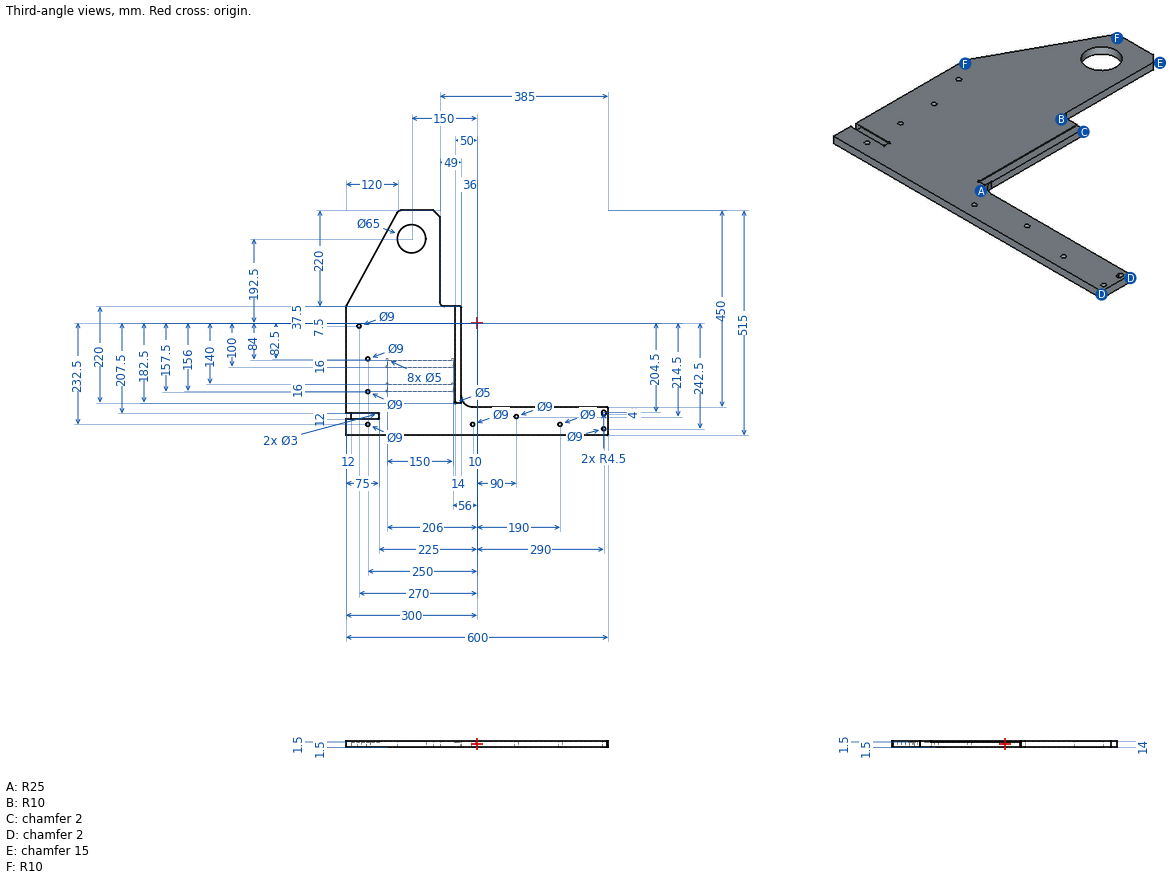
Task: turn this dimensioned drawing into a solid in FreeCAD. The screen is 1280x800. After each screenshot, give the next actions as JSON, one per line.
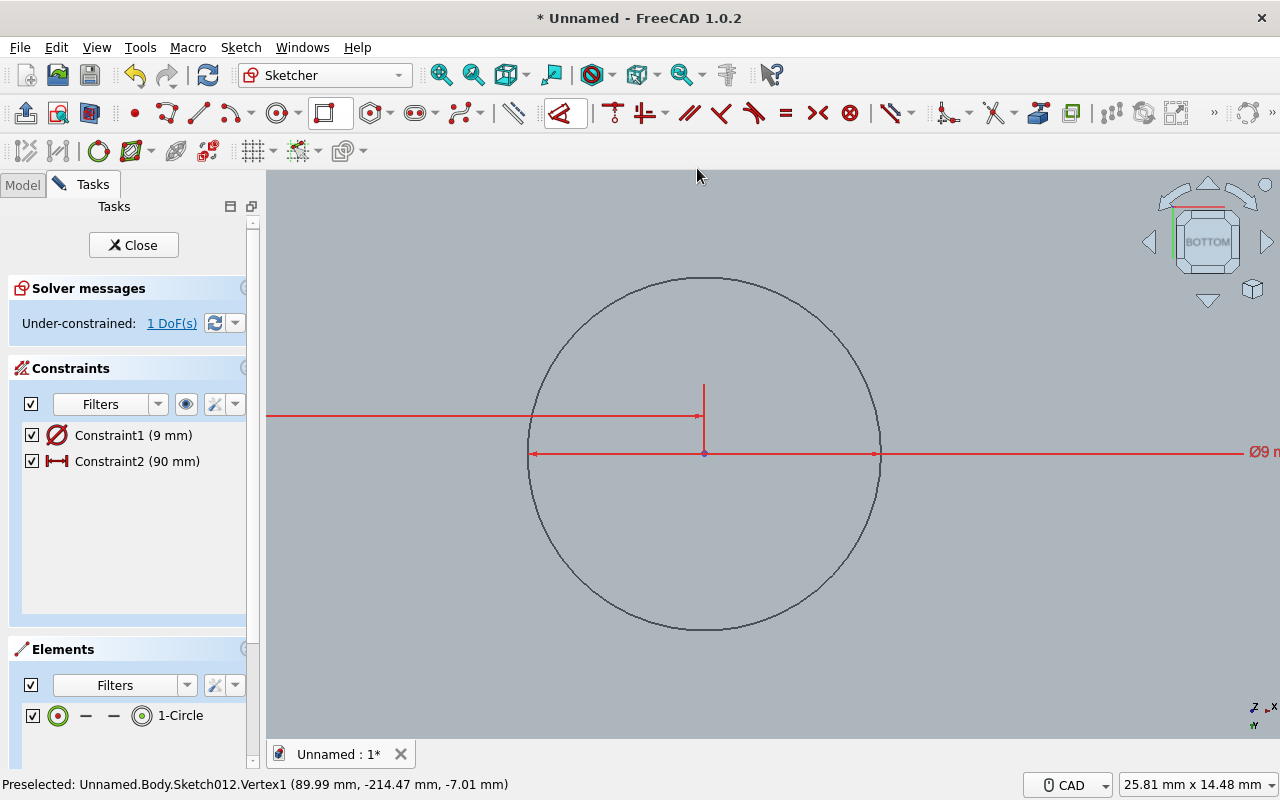
{"action": "left_click", "coordinate": [704, 454]}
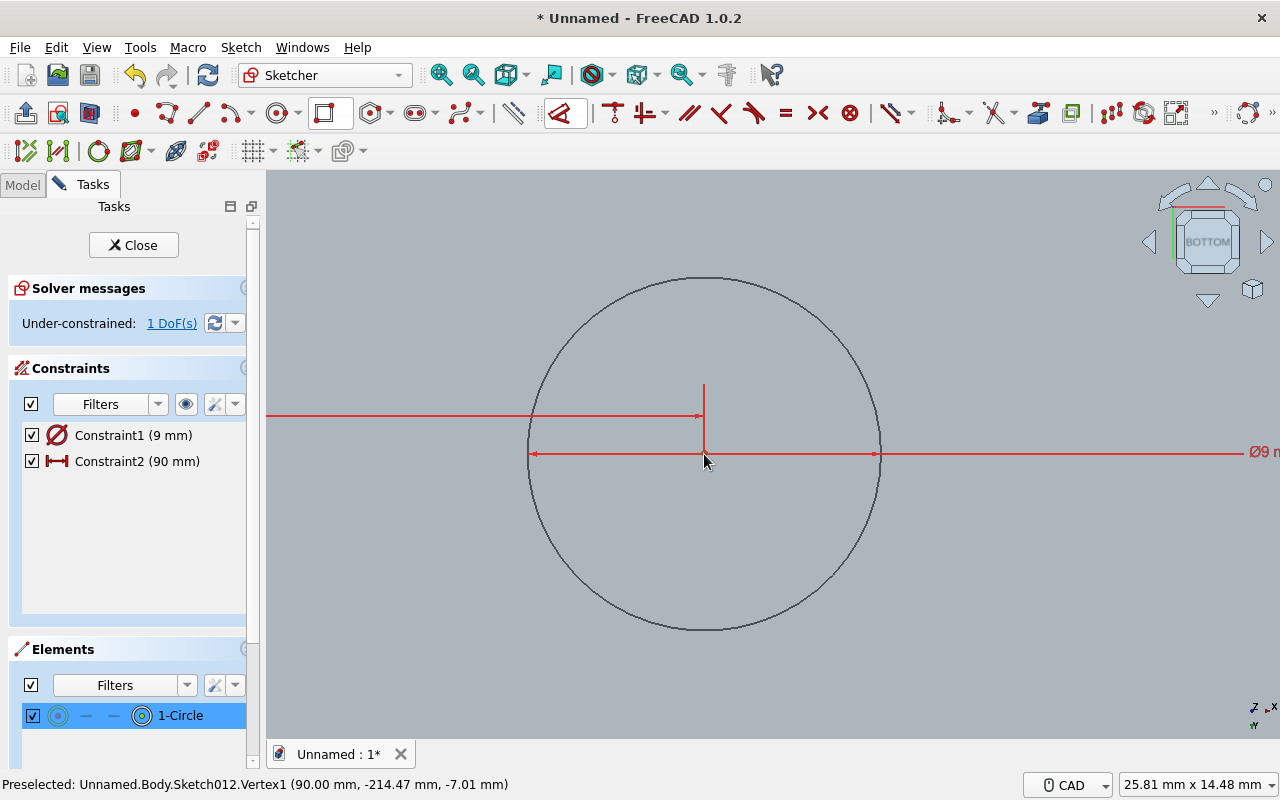
{"action": "left_click", "coordinate": [582, 114]}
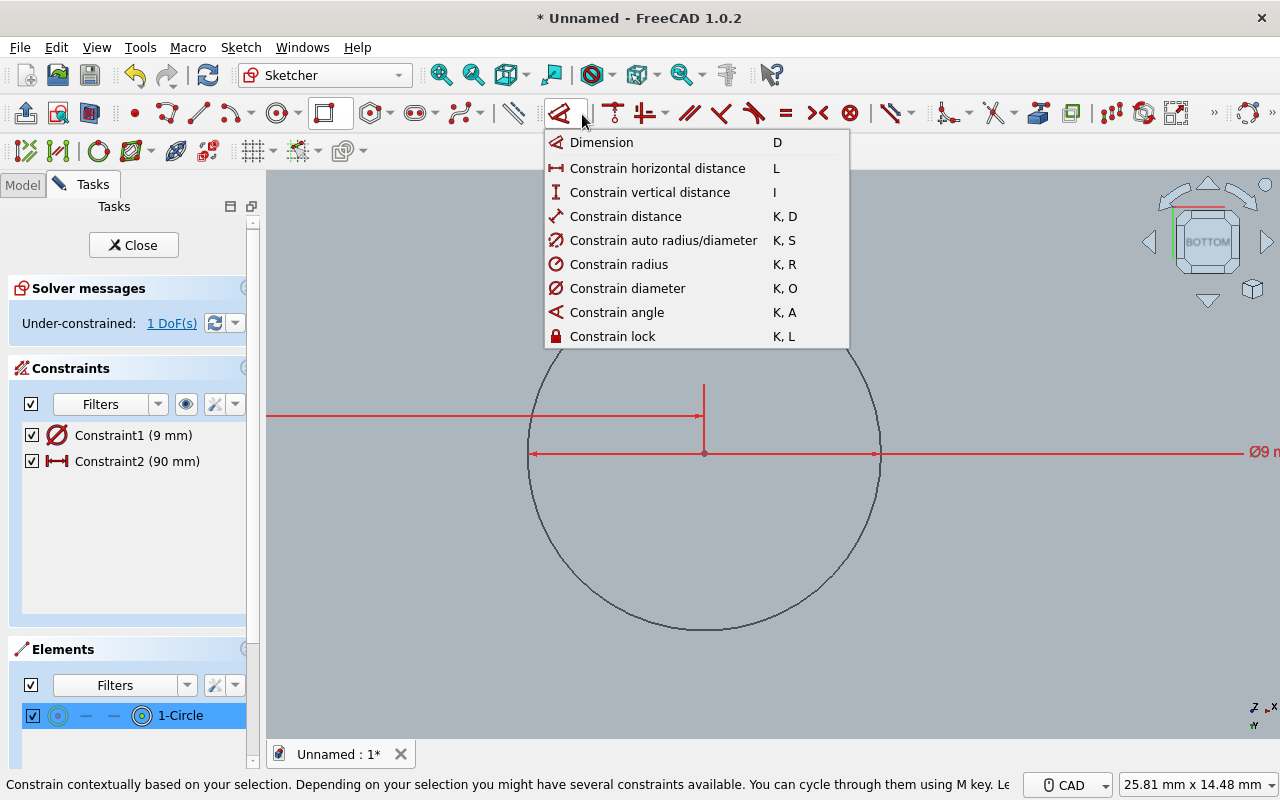
{"action": "left_click", "coordinate": [697, 192]}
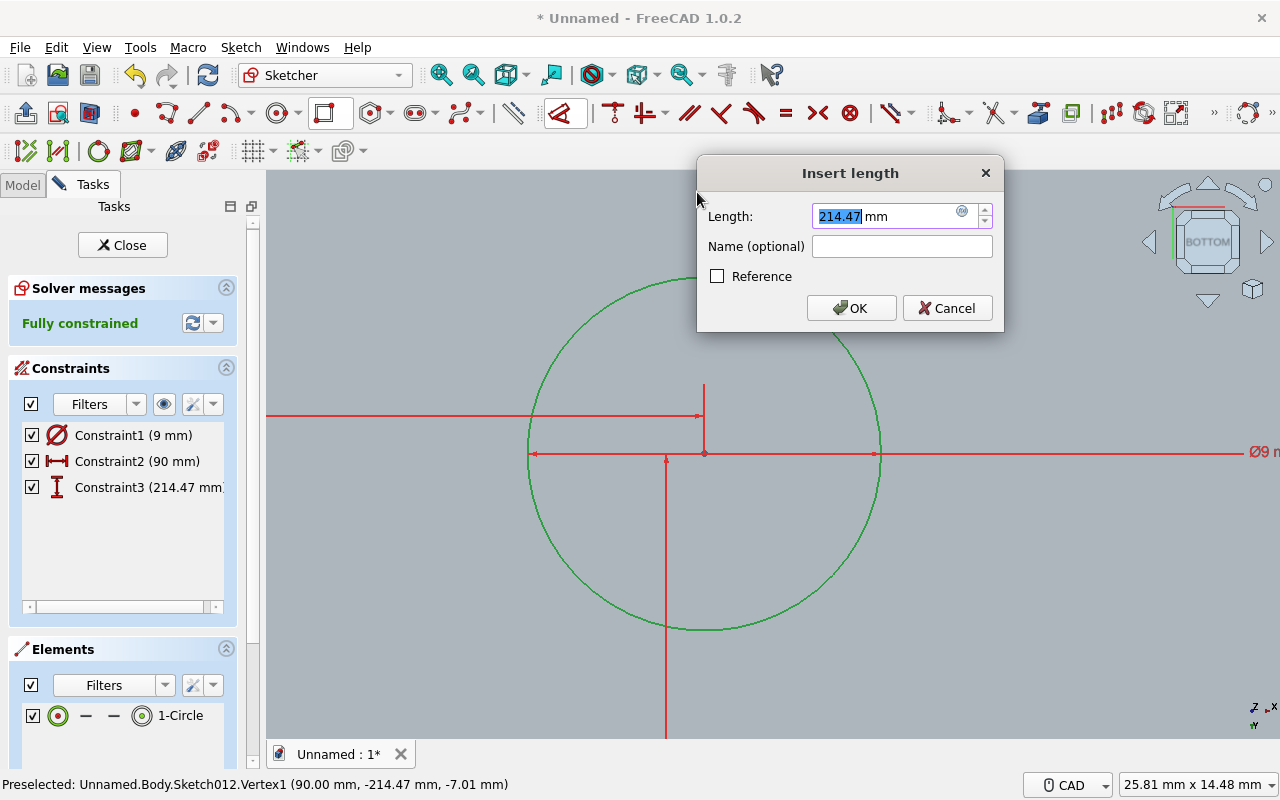
{"action": "type", "text": "214.5"}
{"action": "key", "text": "Return"}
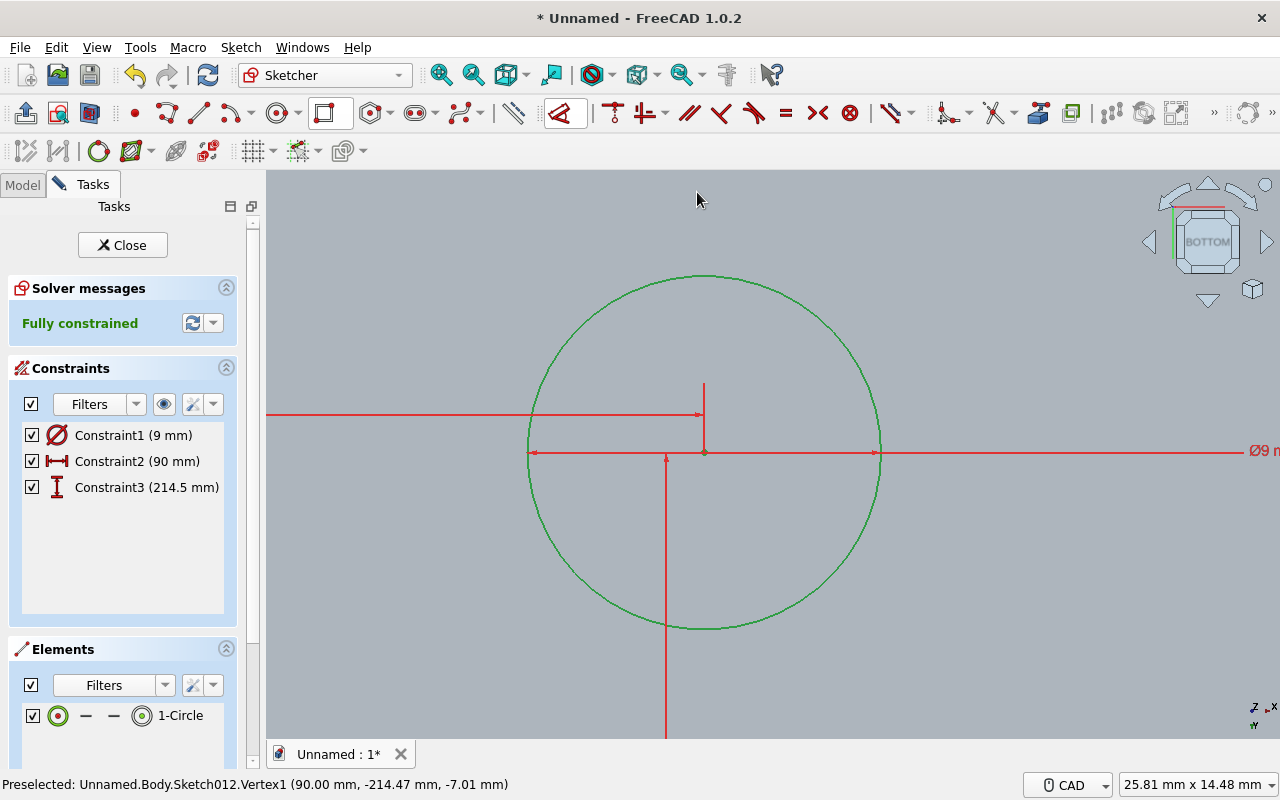
{"action": "left_click", "coordinate": [123, 245]}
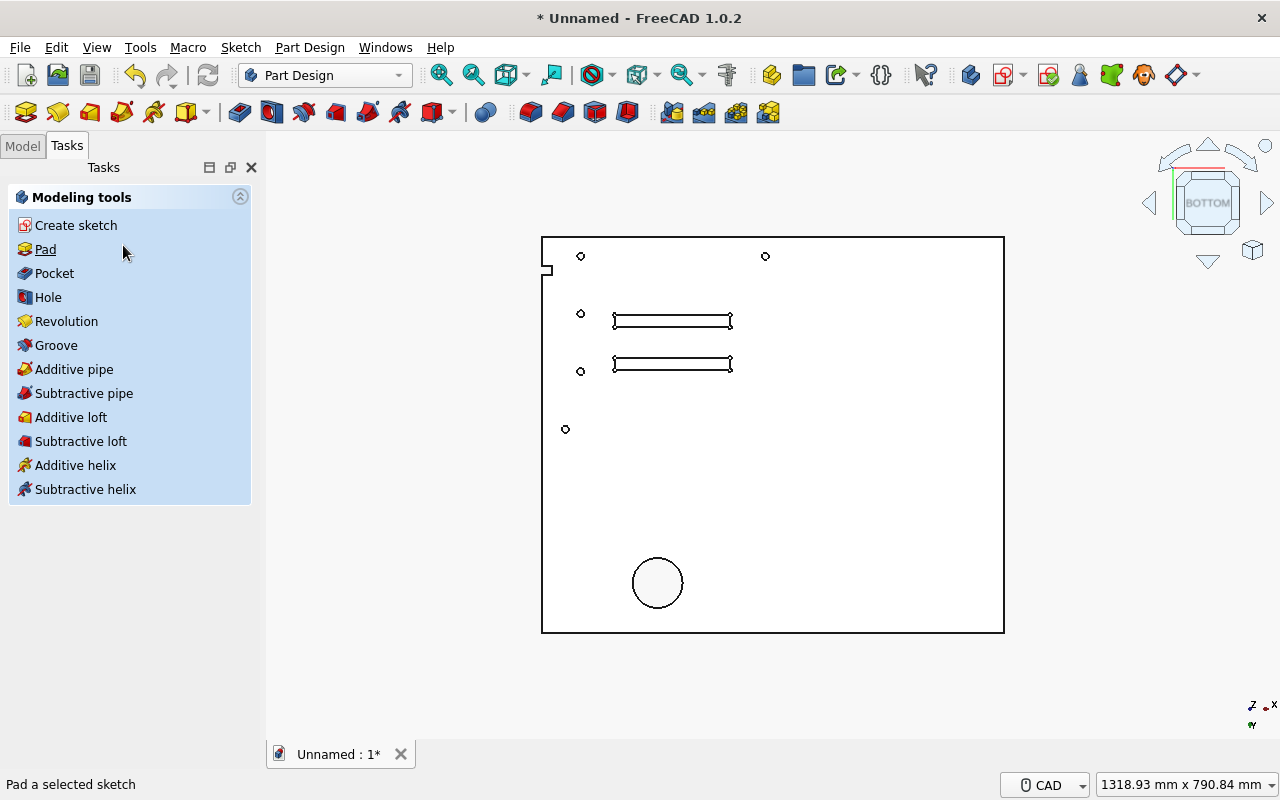
{"action": "left_click", "coordinate": [240, 112]}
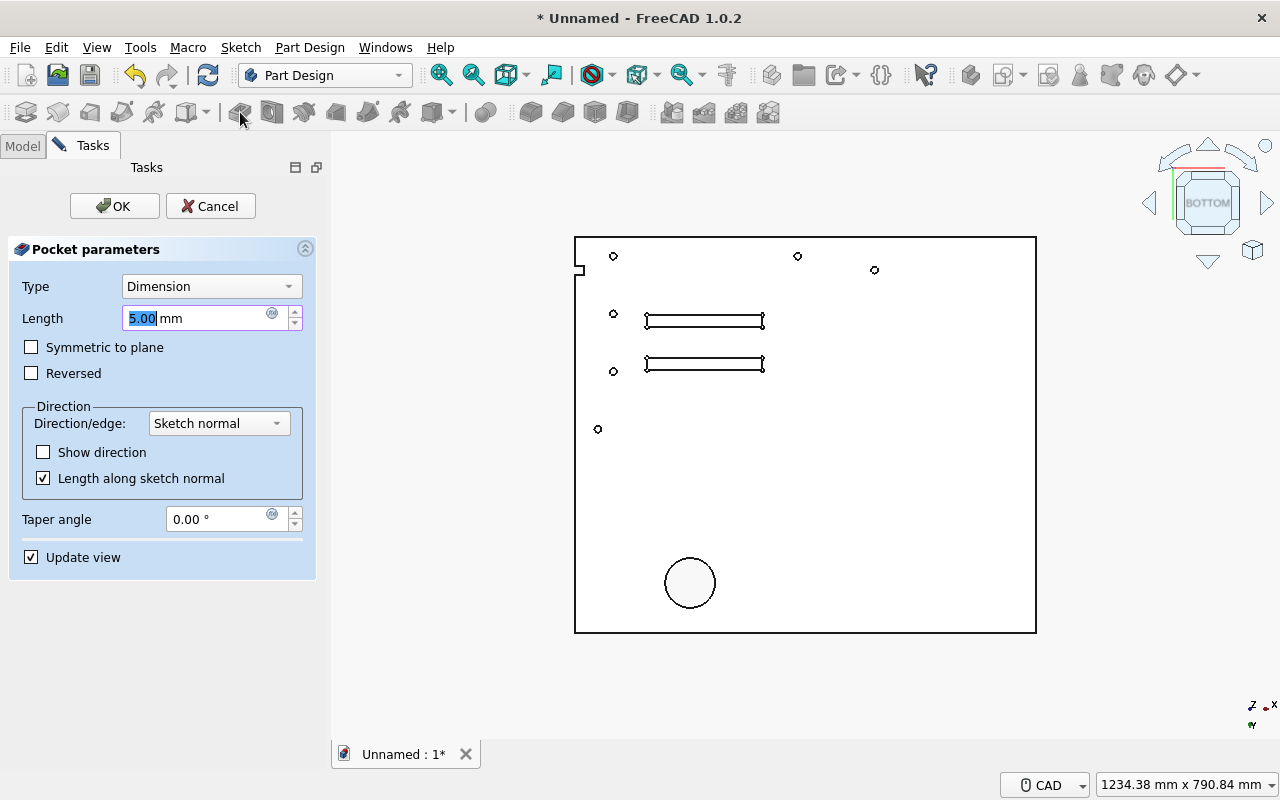
{"action": "left_click", "coordinate": [212, 286]}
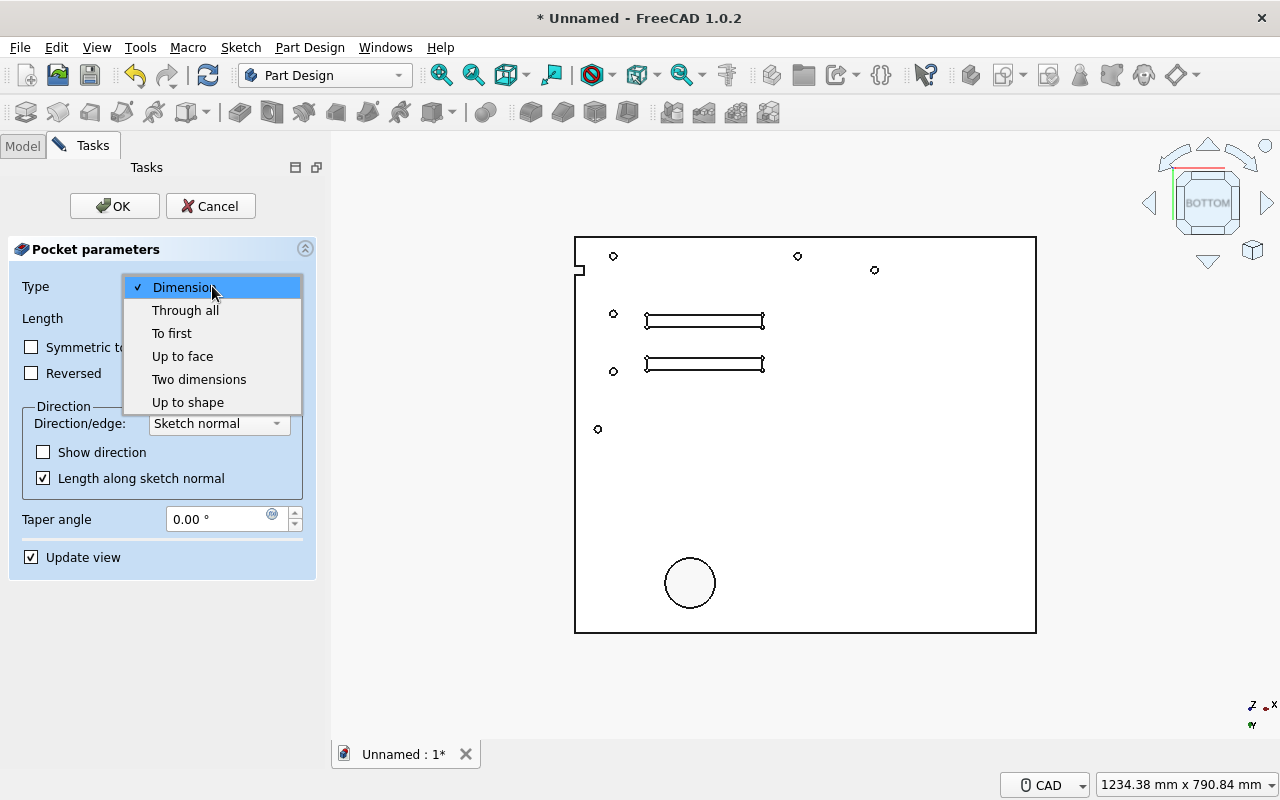
{"action": "left_click", "coordinate": [212, 334]}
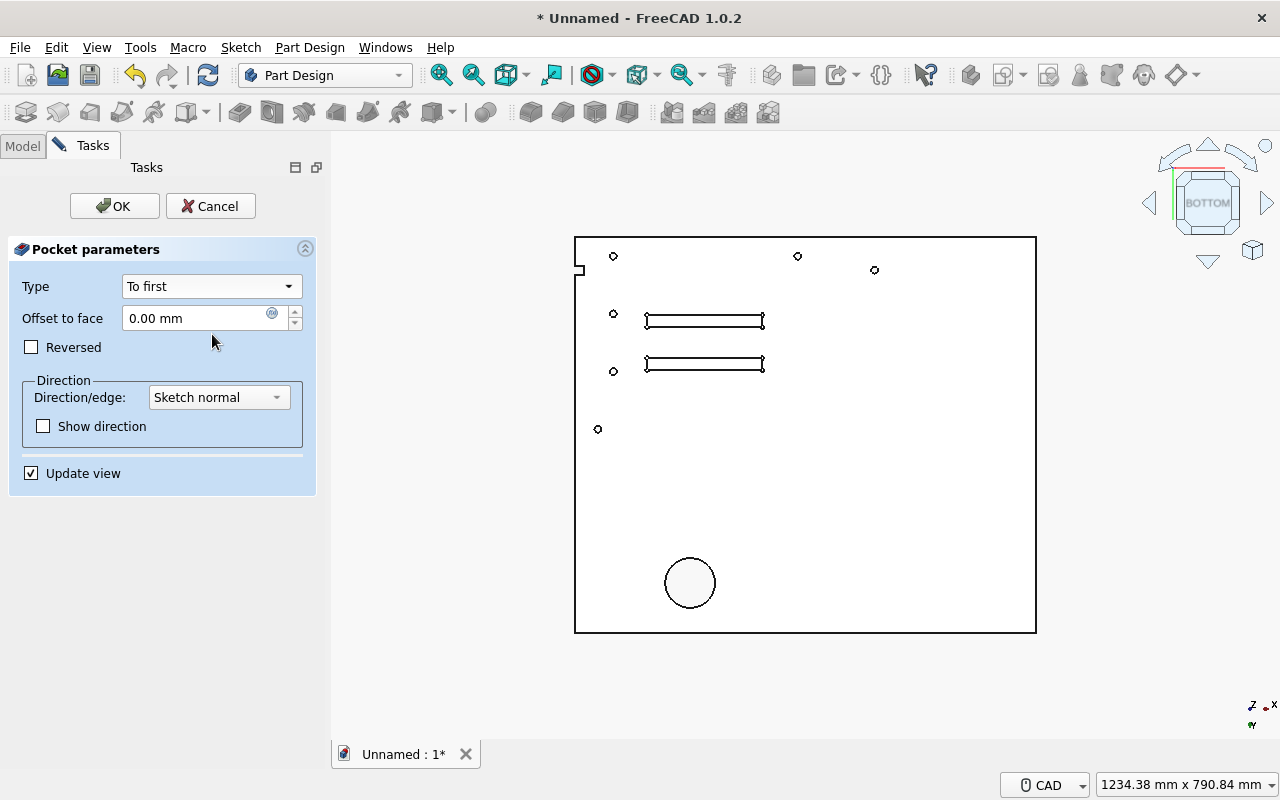
{"action": "left_click", "coordinate": [115, 206]}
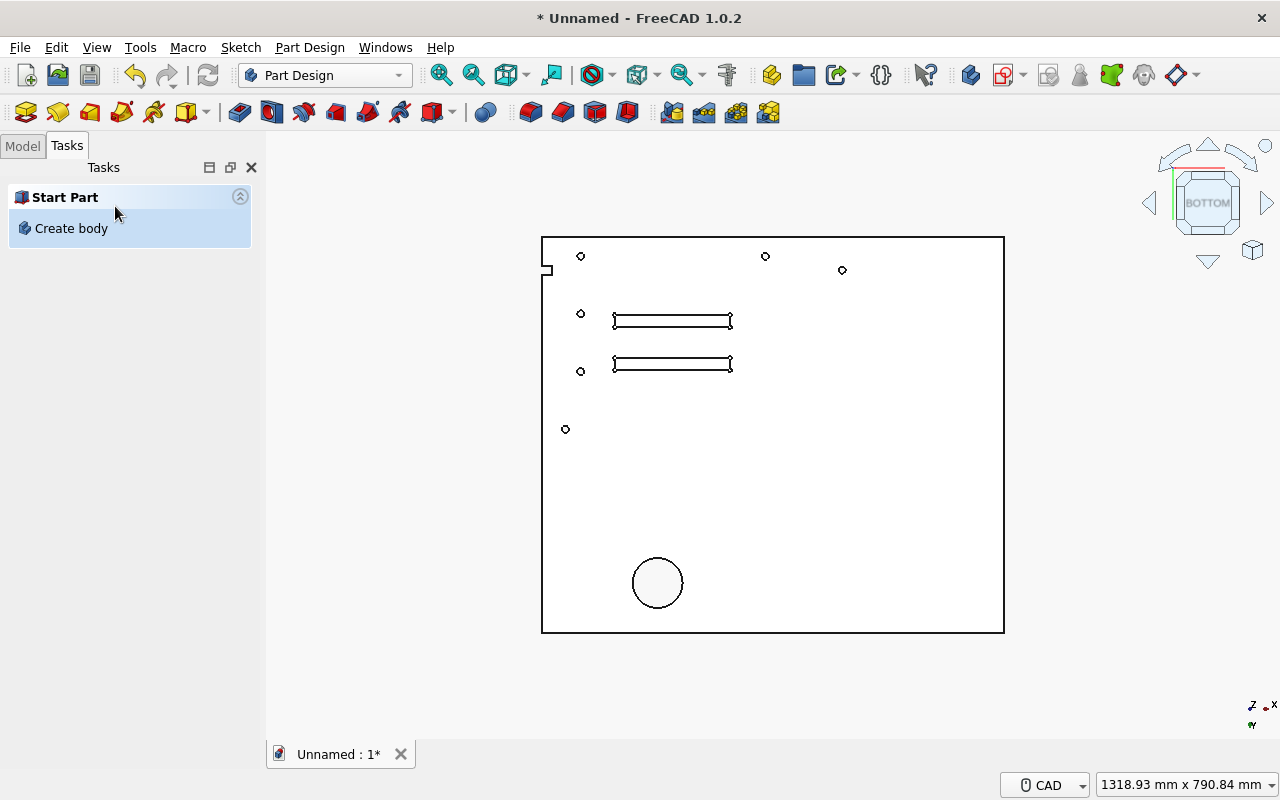
{"action": "left_click", "coordinate": [839, 491]}